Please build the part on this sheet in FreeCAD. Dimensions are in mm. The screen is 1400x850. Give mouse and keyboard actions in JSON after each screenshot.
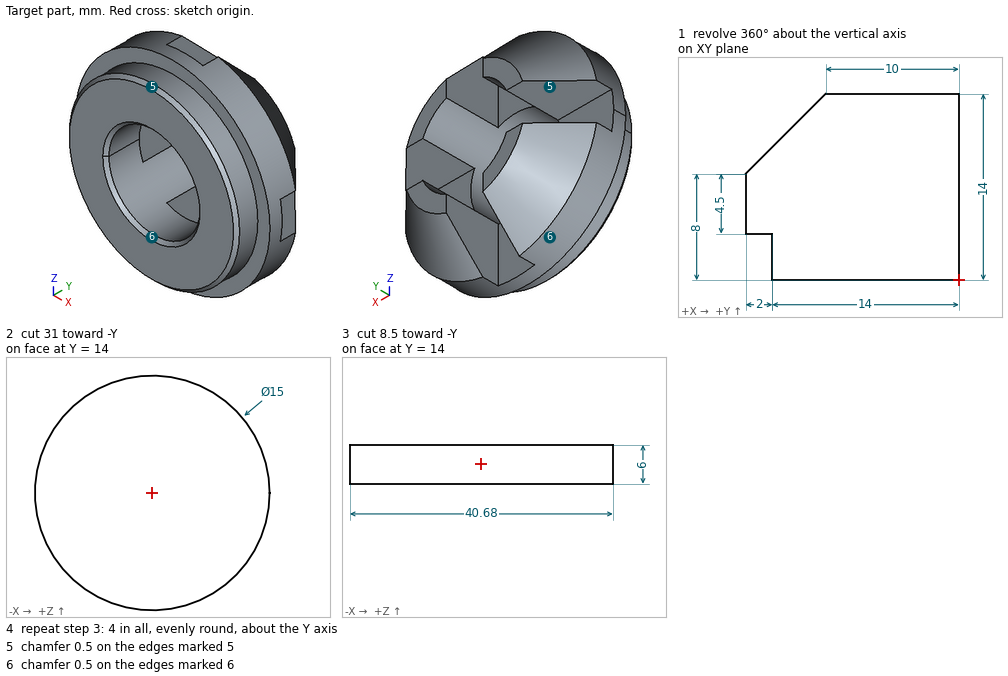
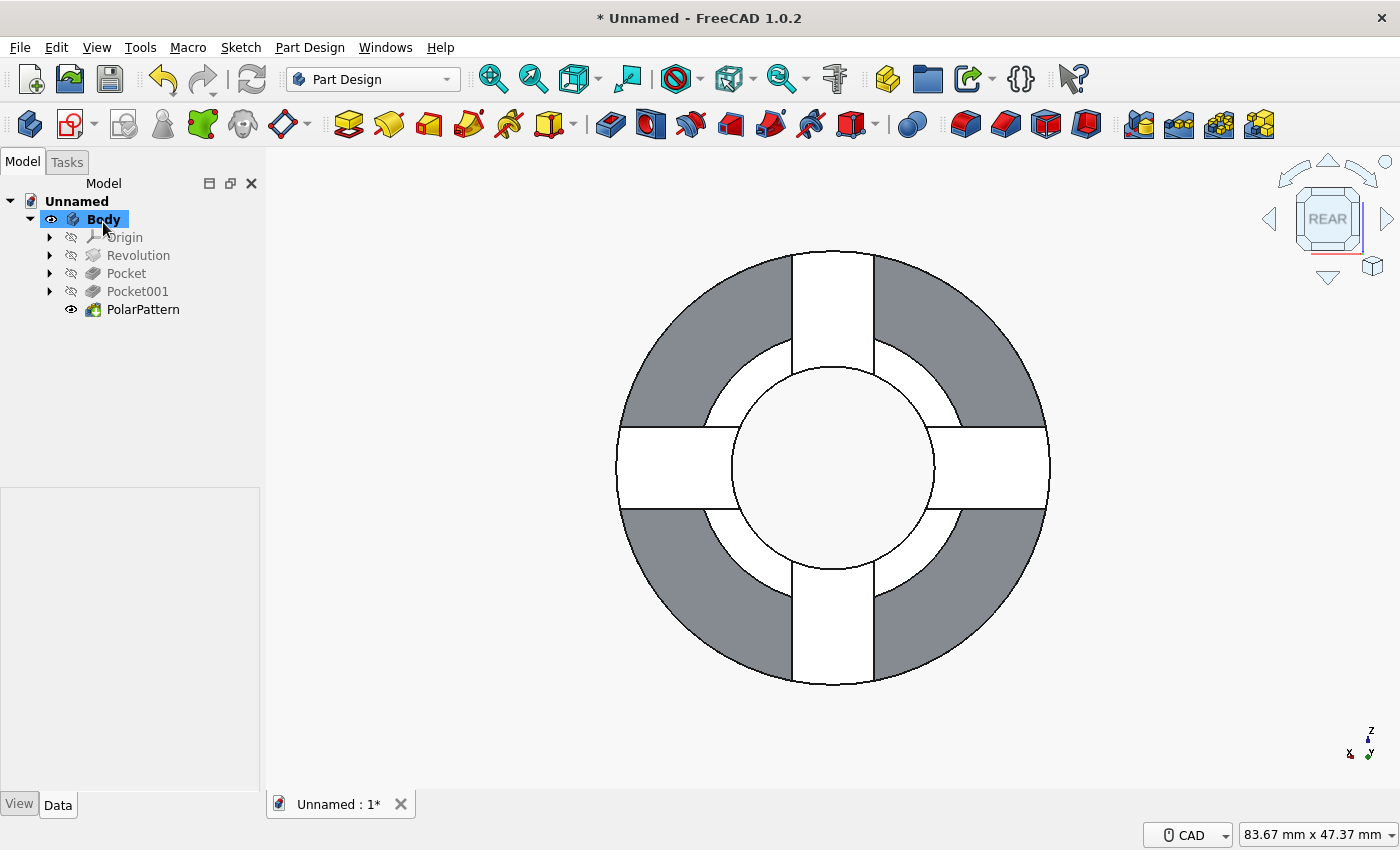
{"action": "key", "text": "0"}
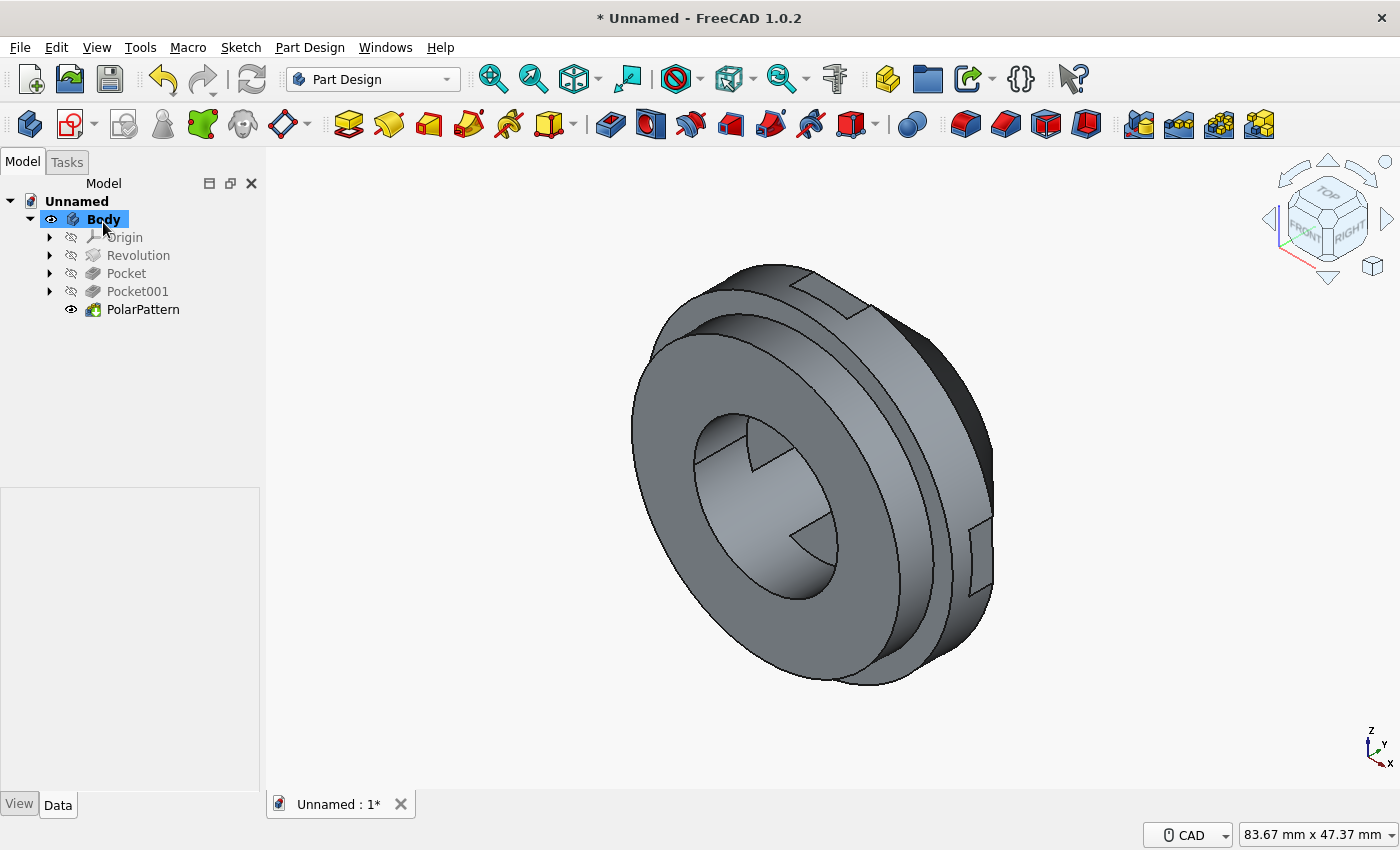
{"action": "left_click", "coordinate": [900, 583]}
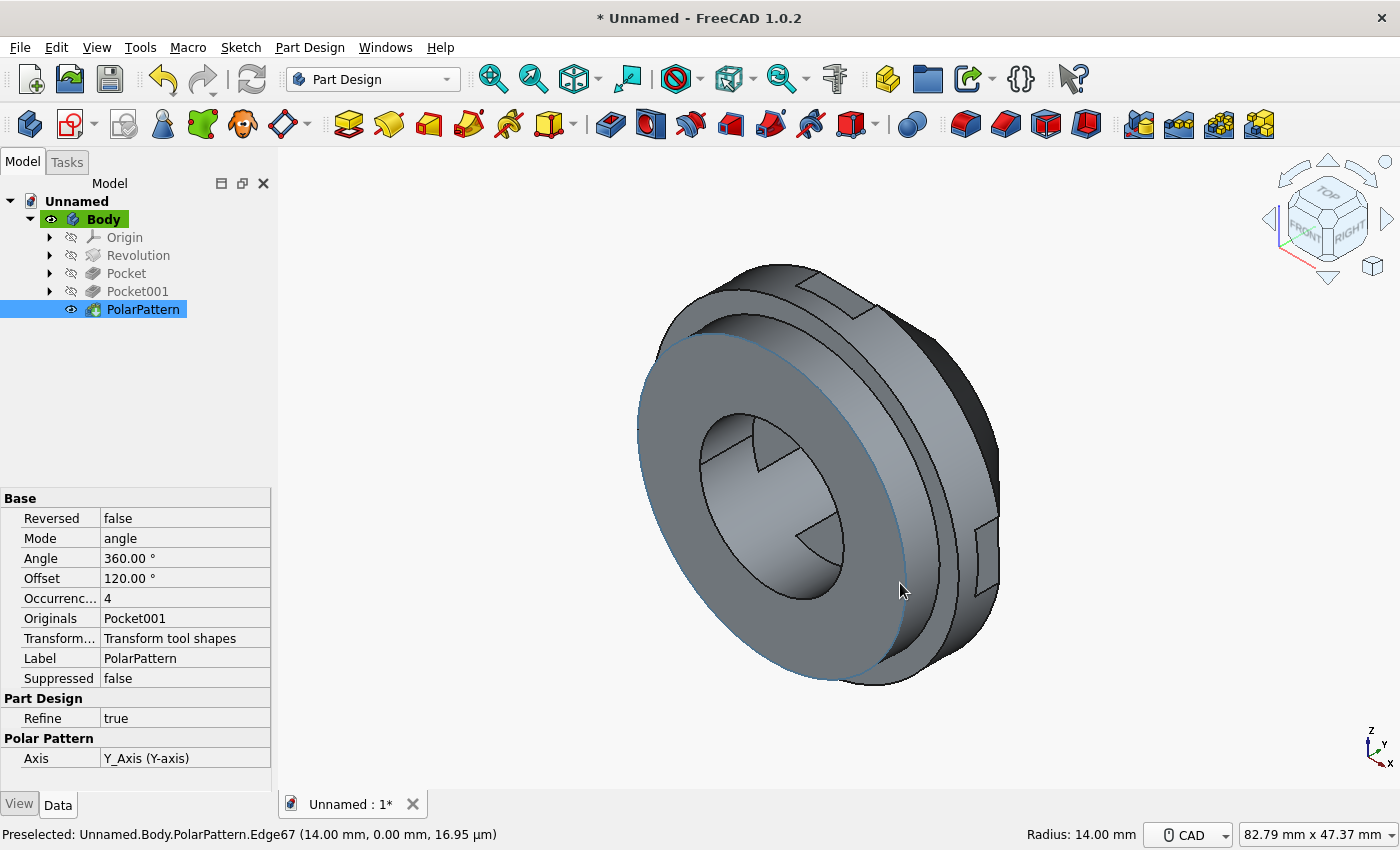
{"action": "left_click", "coordinate": [1006, 124]}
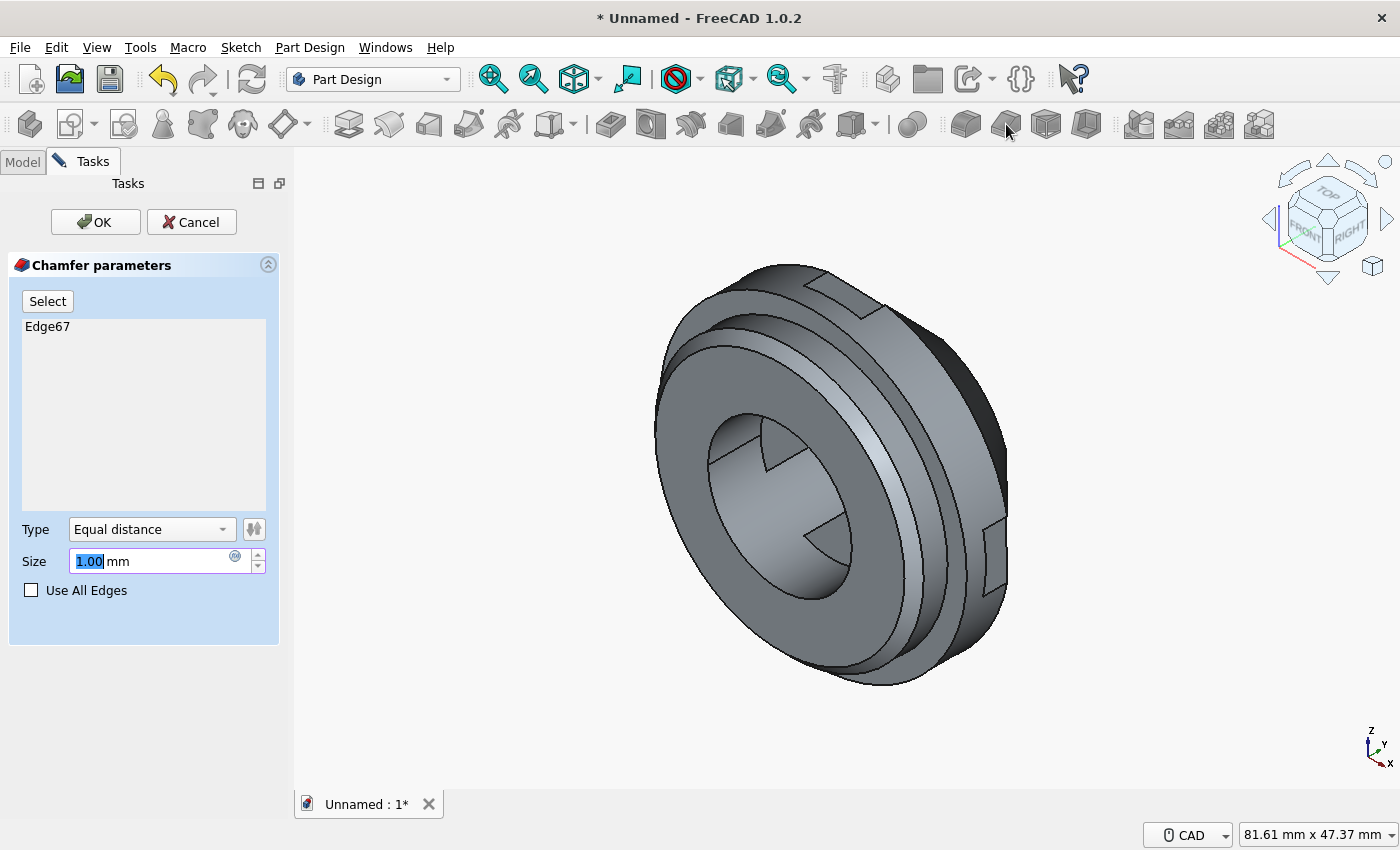
{"action": "type", "text": "0.5"}
{"action": "key", "text": "Tab"}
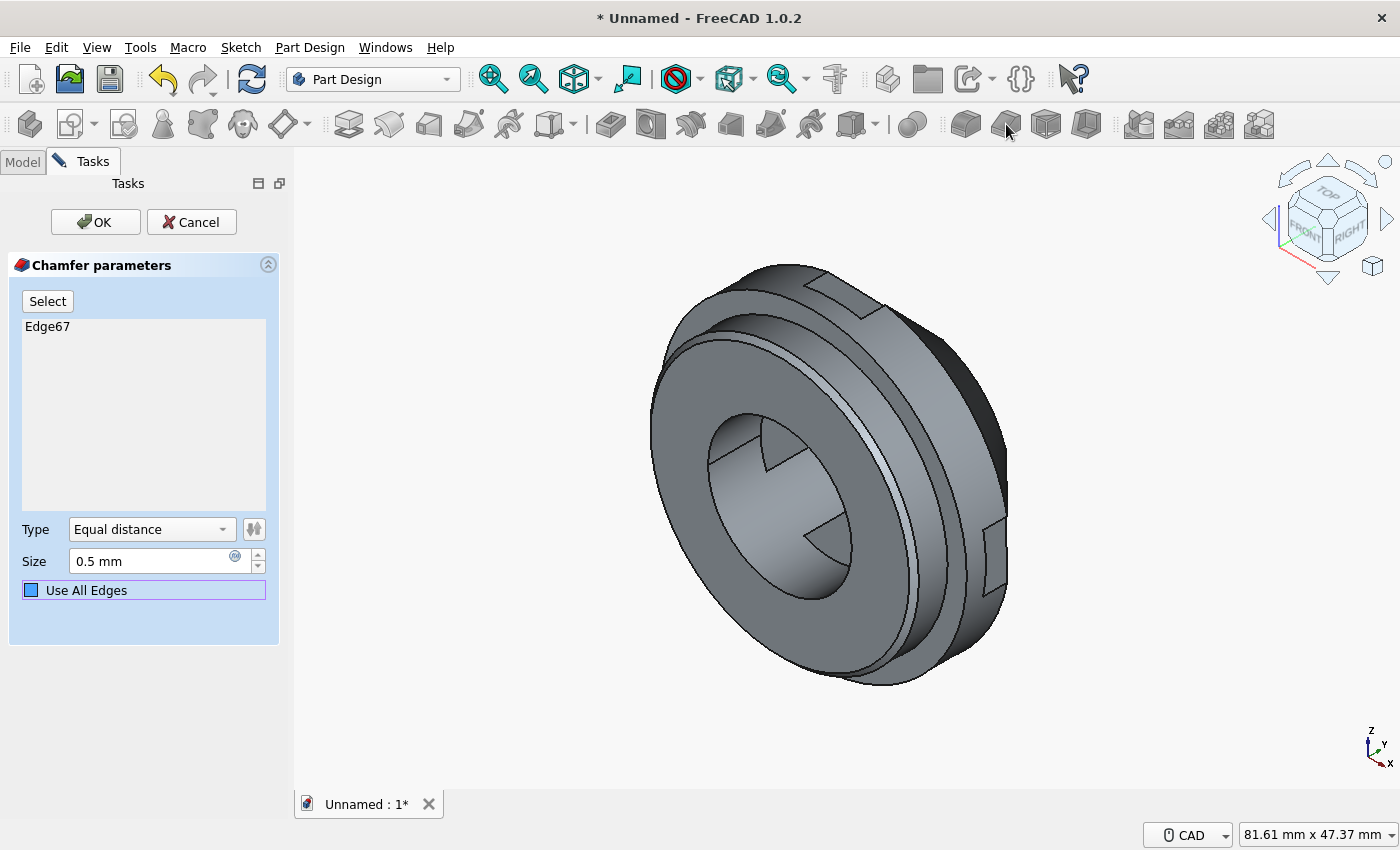
{"action": "left_click", "coordinate": [96, 222]}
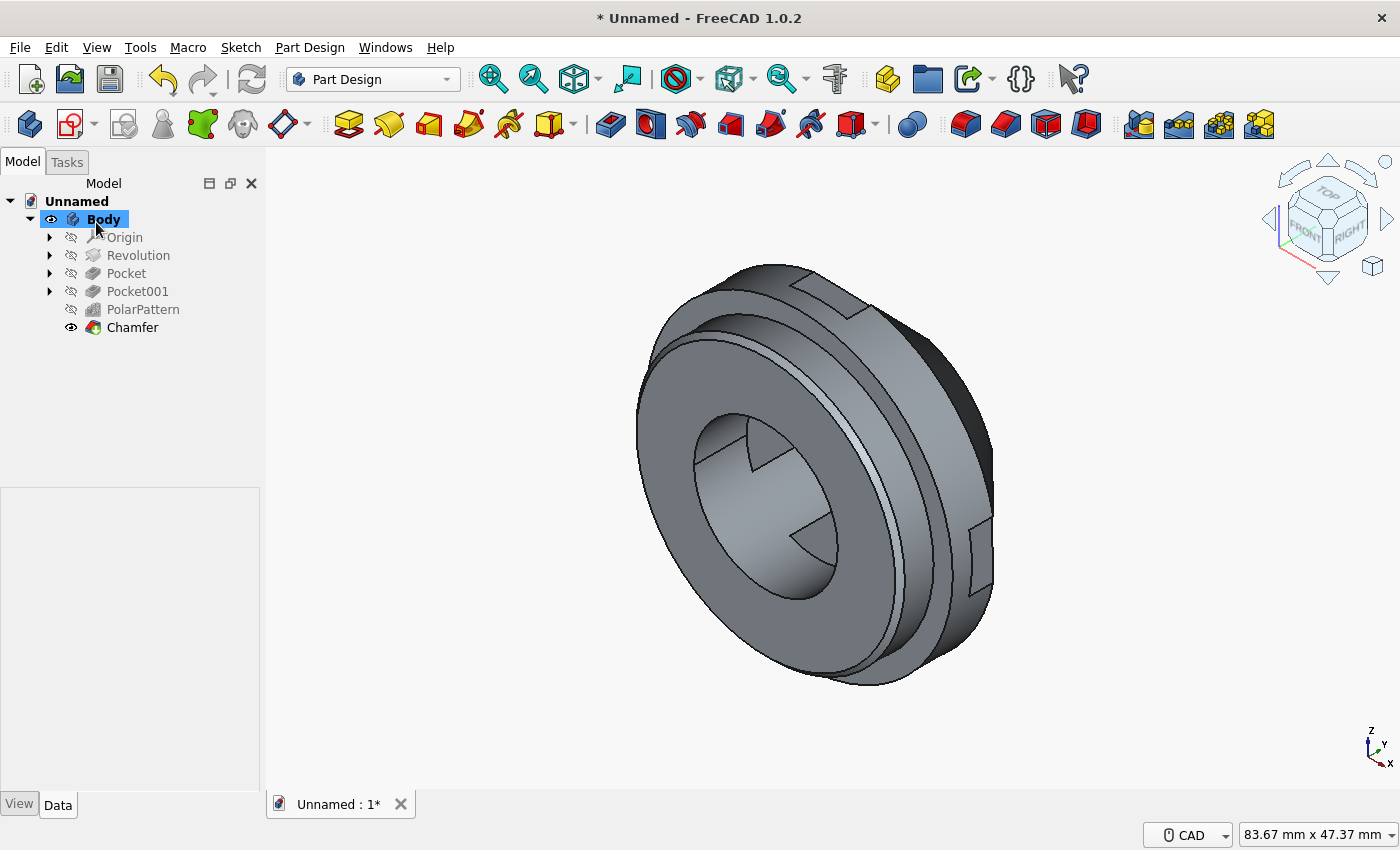
{"action": "left_click", "coordinate": [788, 597]}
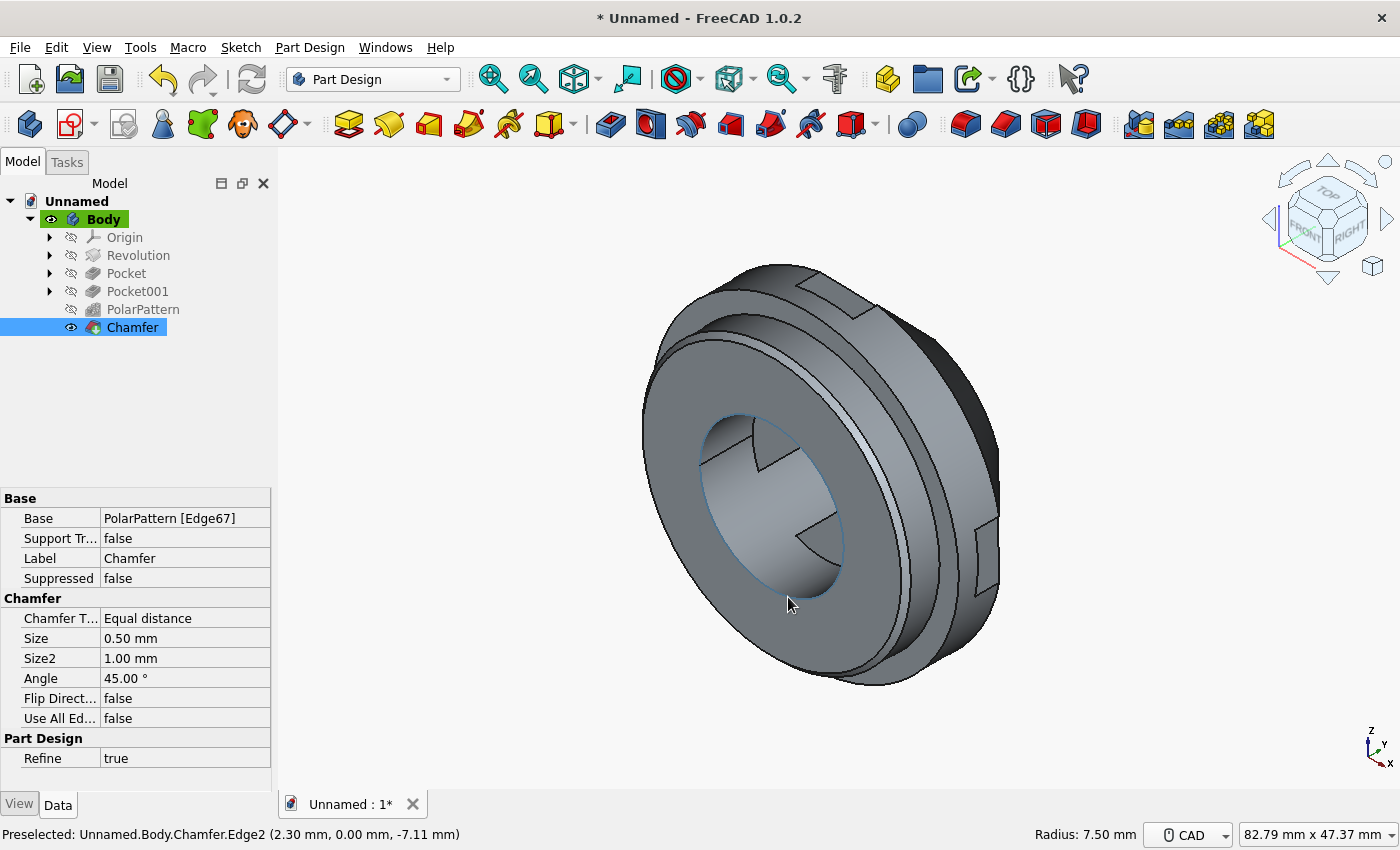
{"action": "left_click", "coordinate": [1006, 124]}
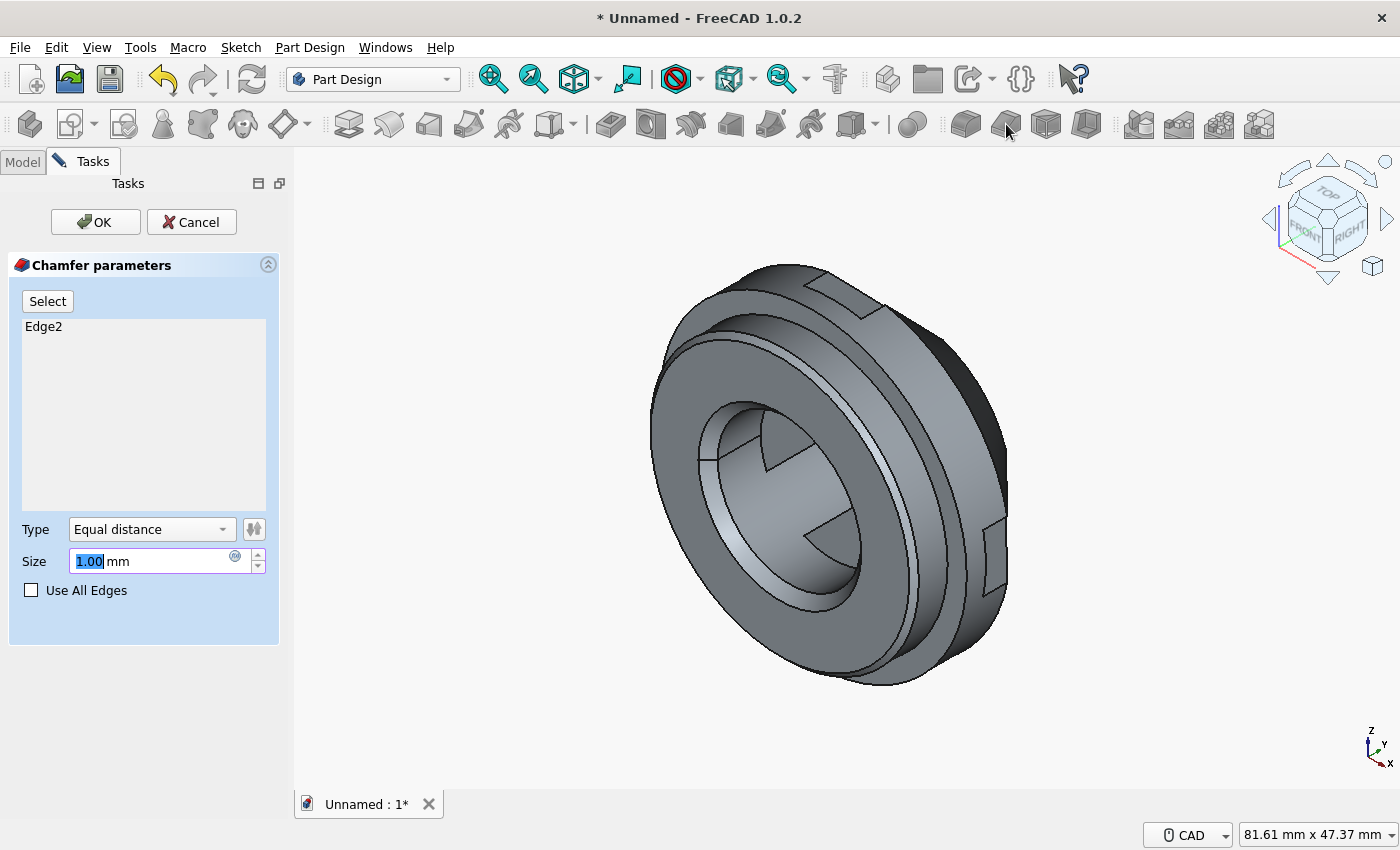
{"action": "type", "text": "0.5"}
{"action": "key", "text": "Tab"}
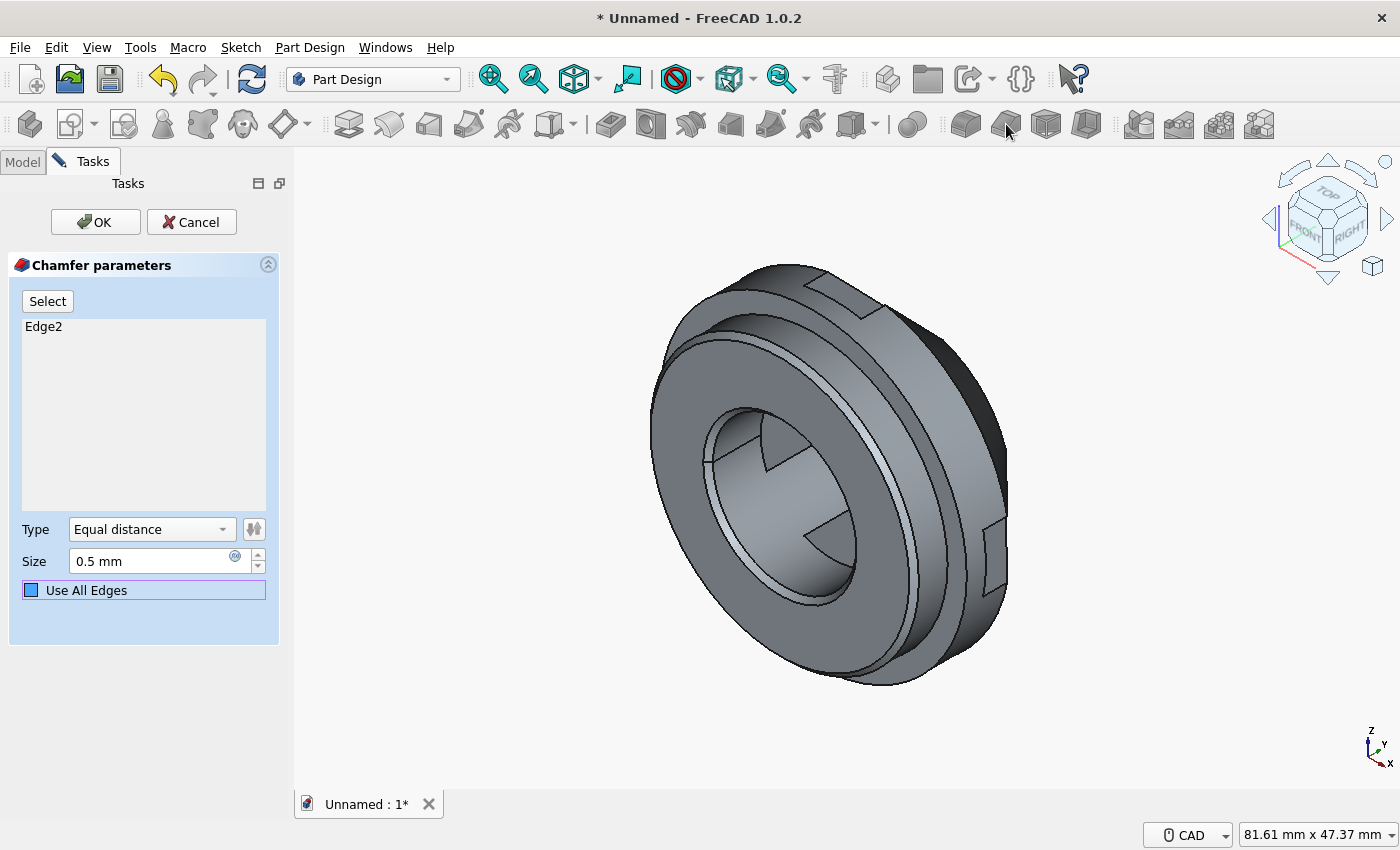
{"action": "left_click", "coordinate": [96, 222]}